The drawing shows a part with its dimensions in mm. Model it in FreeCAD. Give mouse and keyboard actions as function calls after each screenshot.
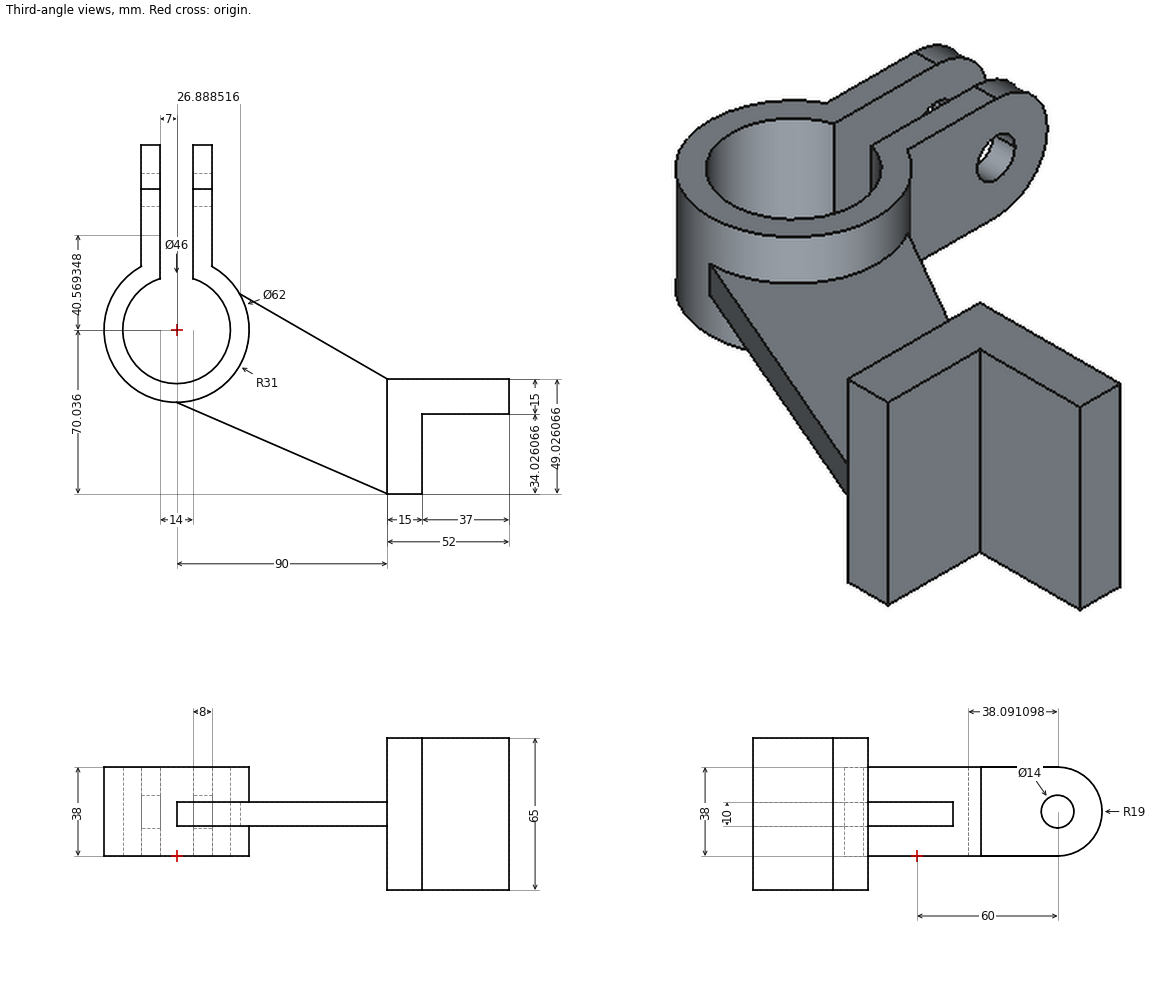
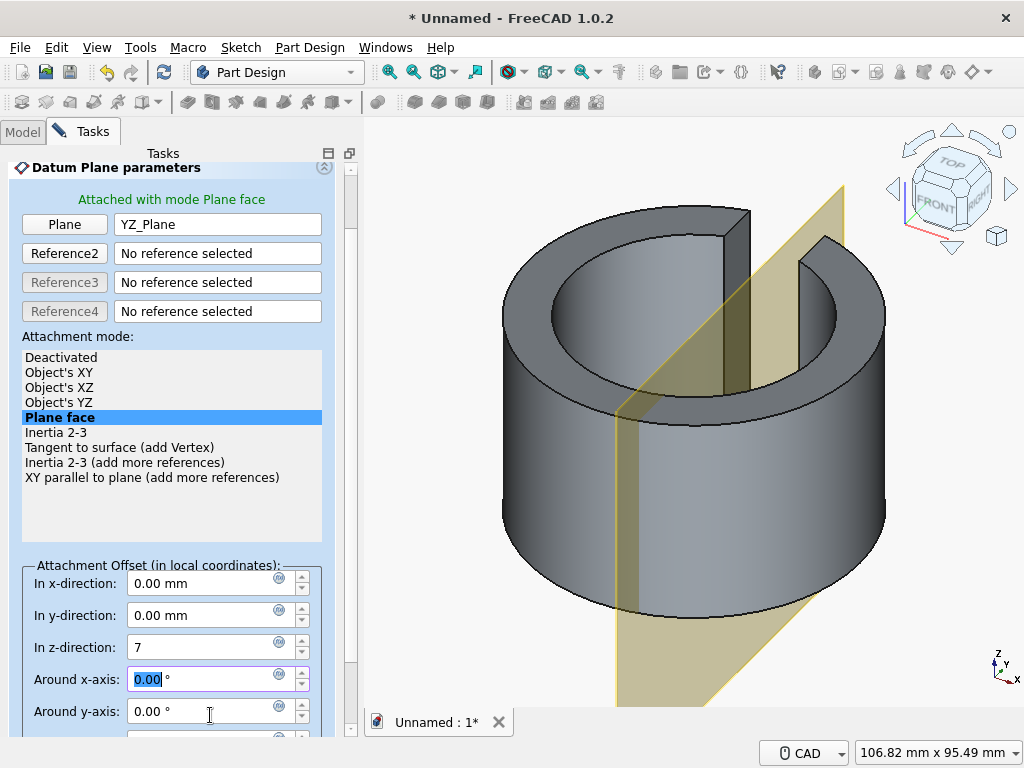
scroll(351, 450, up, 2)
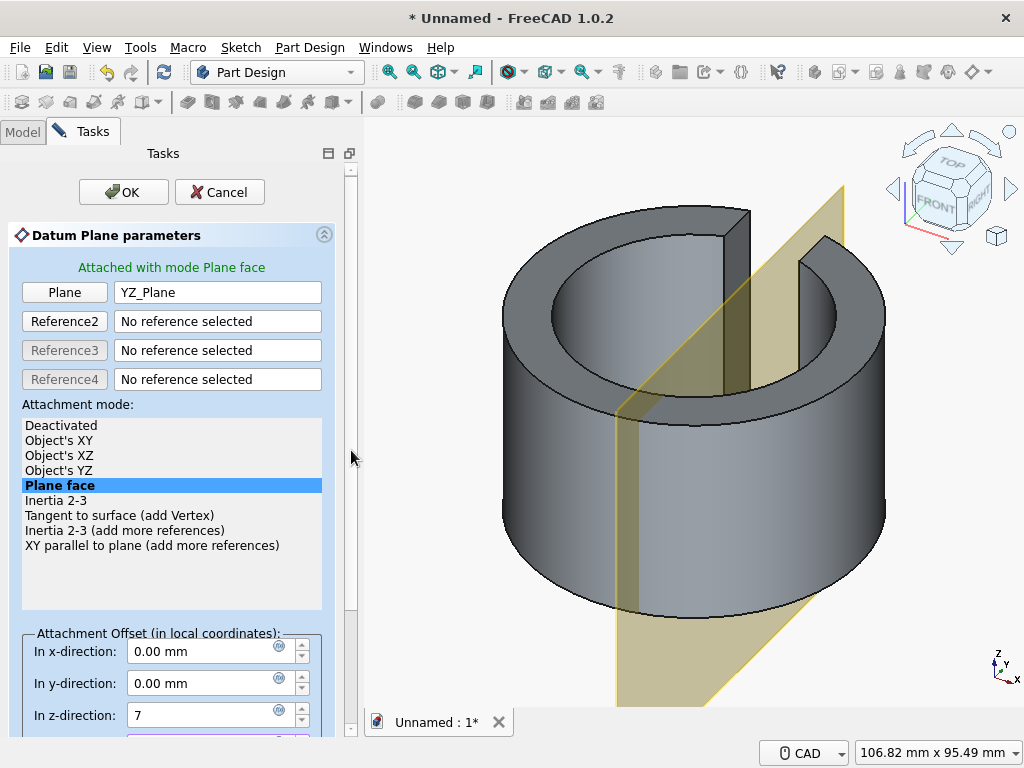
click(124, 192)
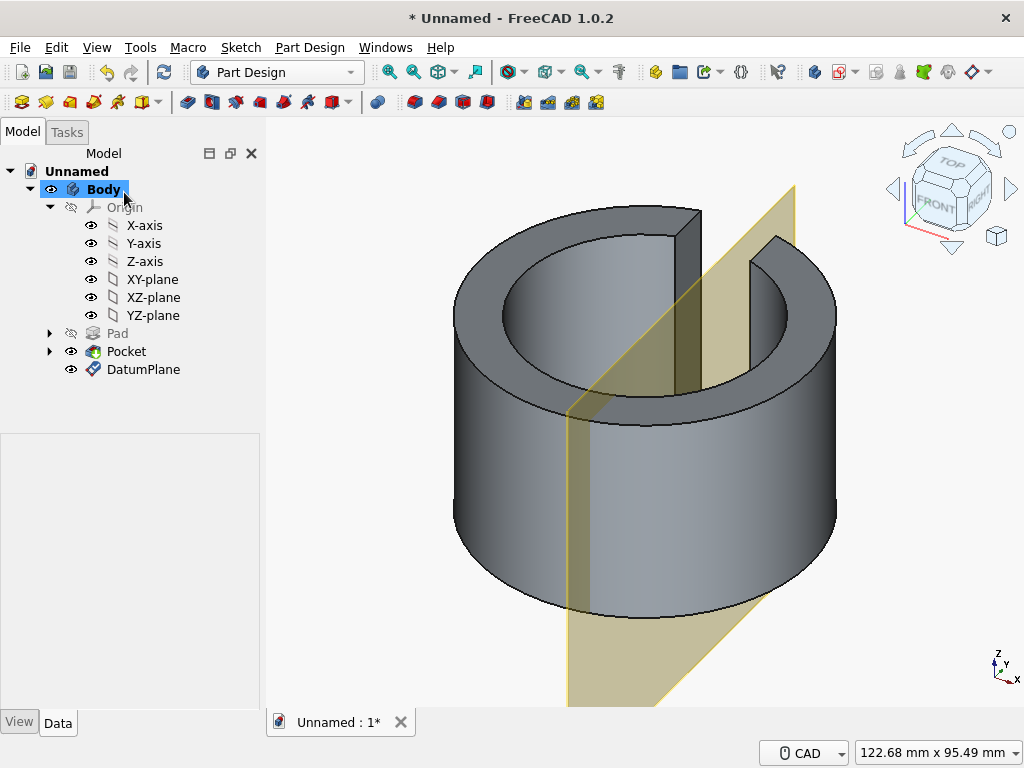
click(116, 369)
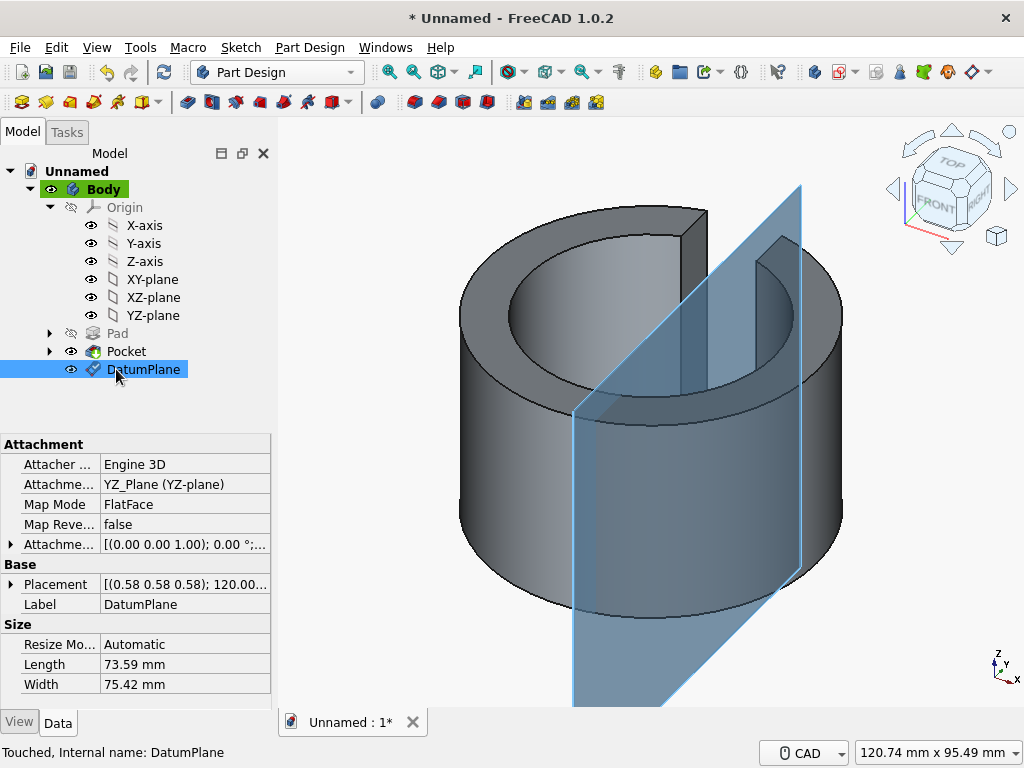
click(840, 72)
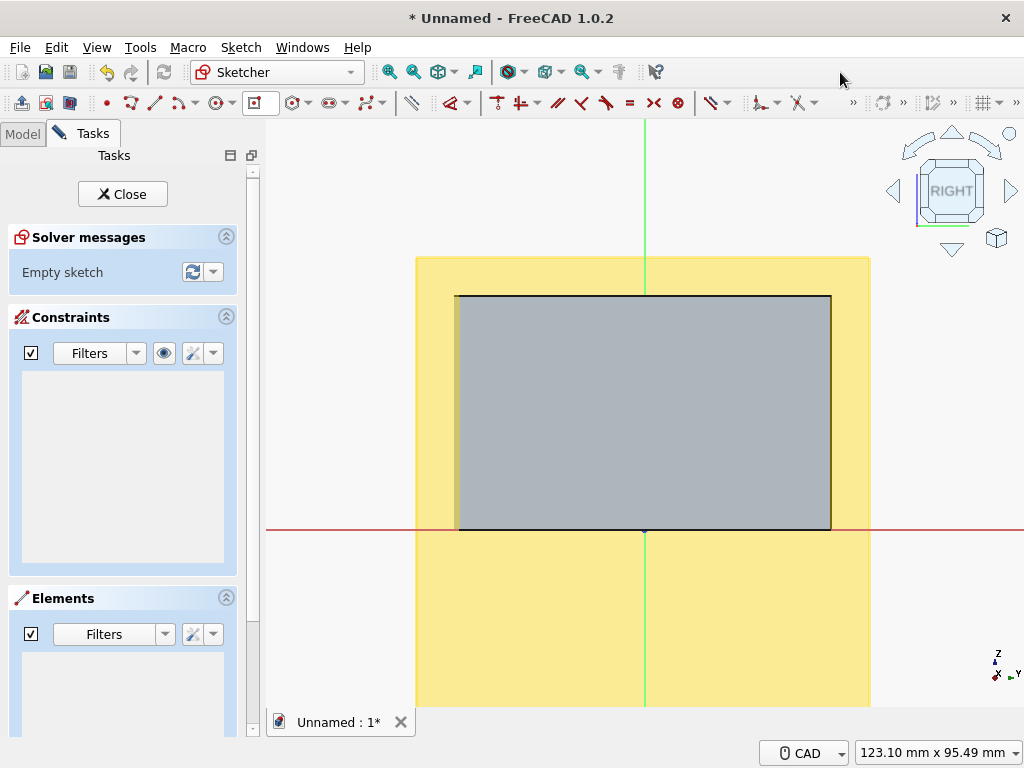
key(q)
key(s)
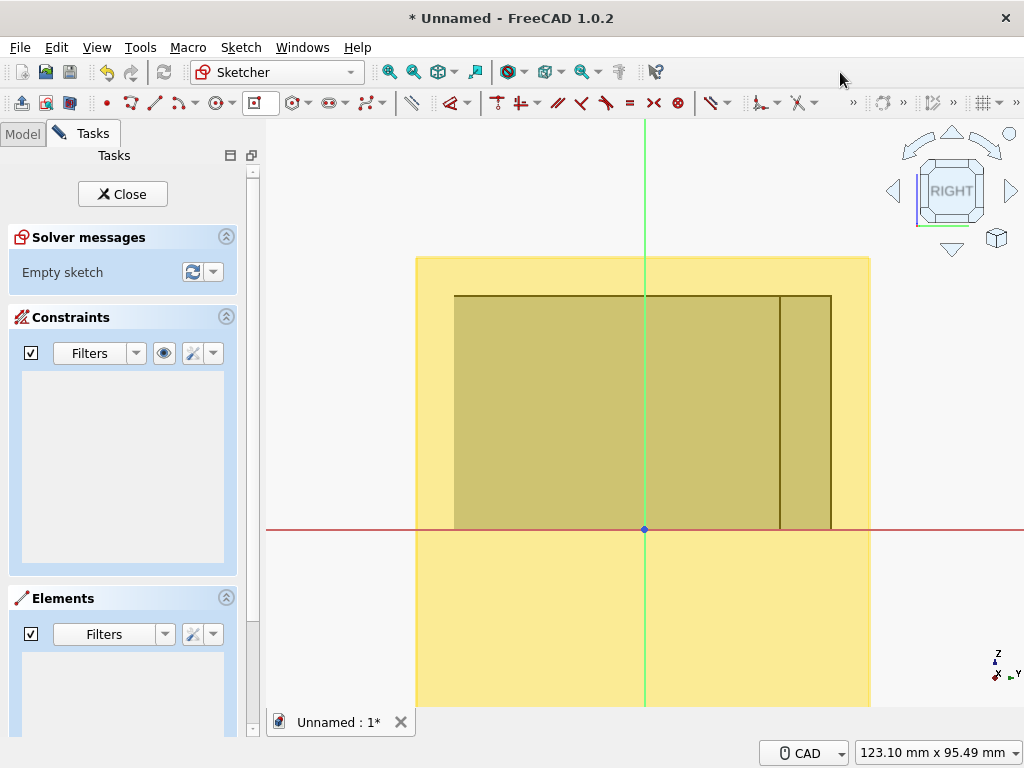
scroll(294, 413, down, 3)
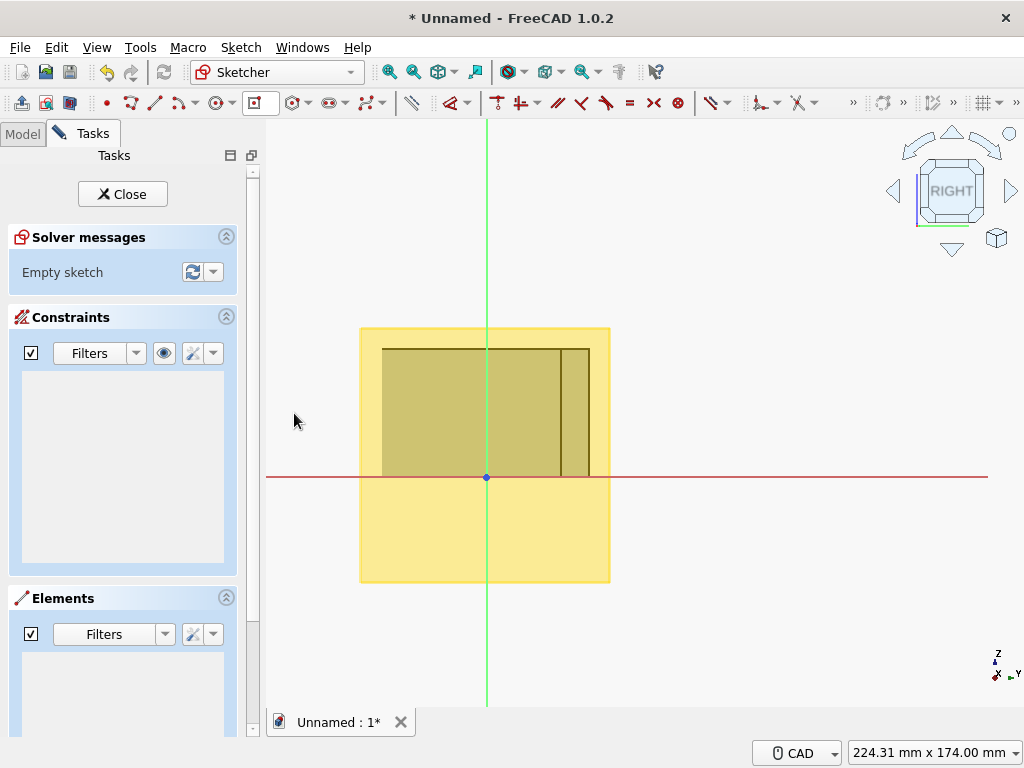
scroll(709, 414, up, 2)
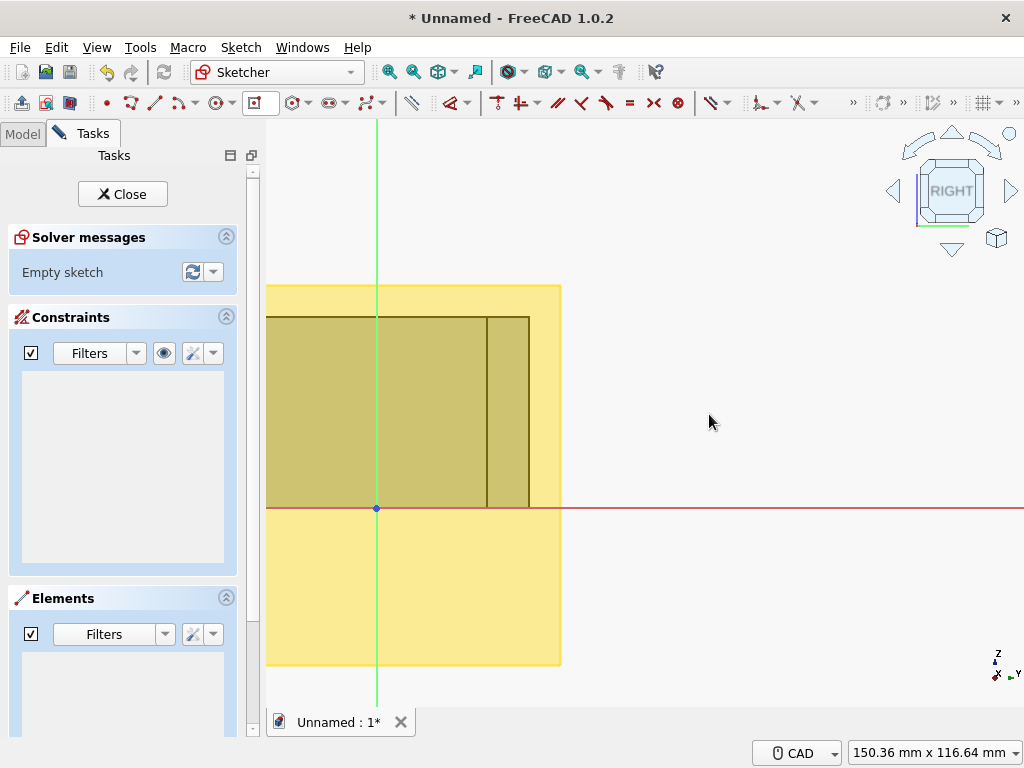
click(132, 104)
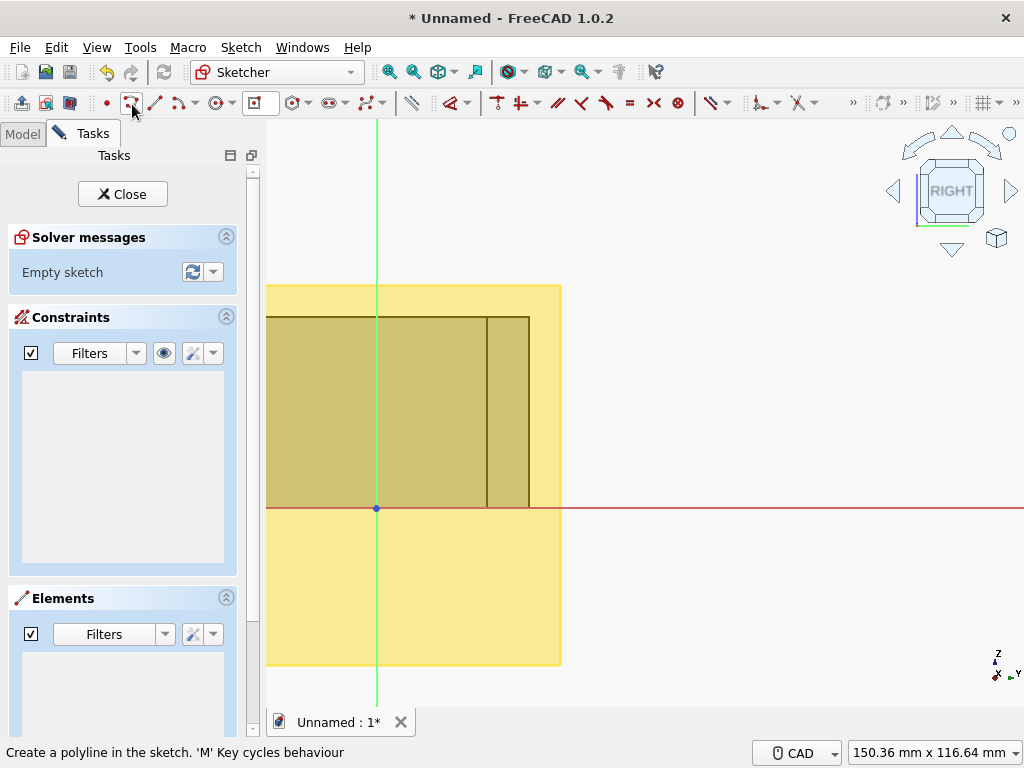
click(679, 317)
click(487, 317)
click(487, 508)
click(679, 499)
right_click(679, 499)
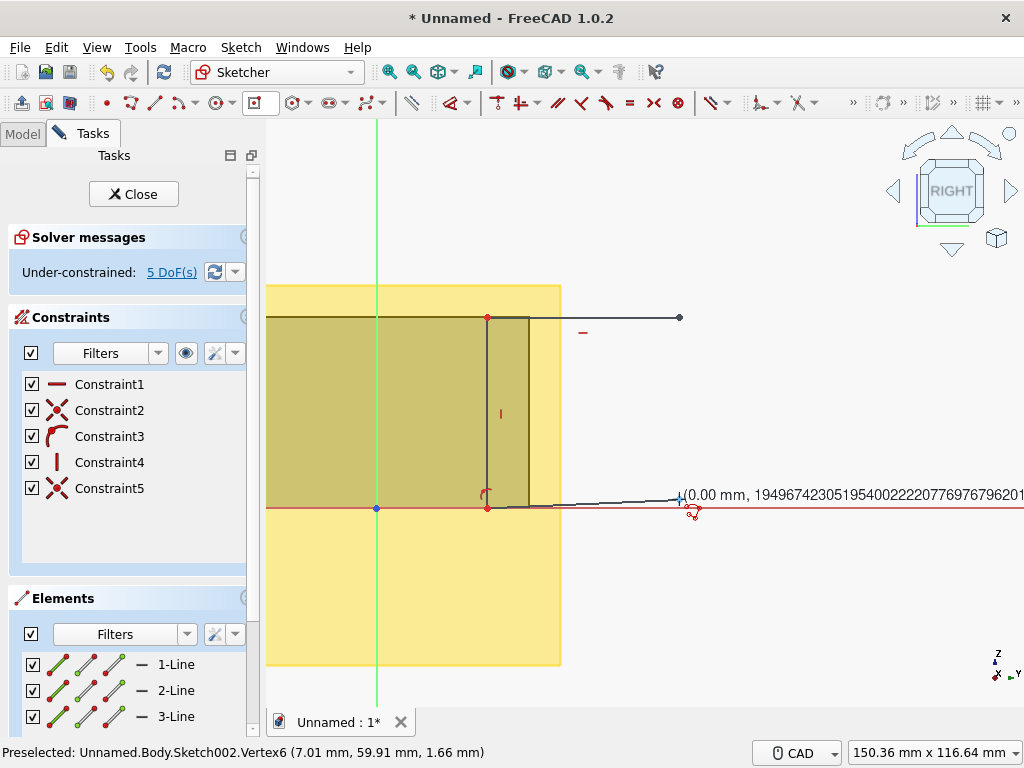
key(g)
key(3)
key(a)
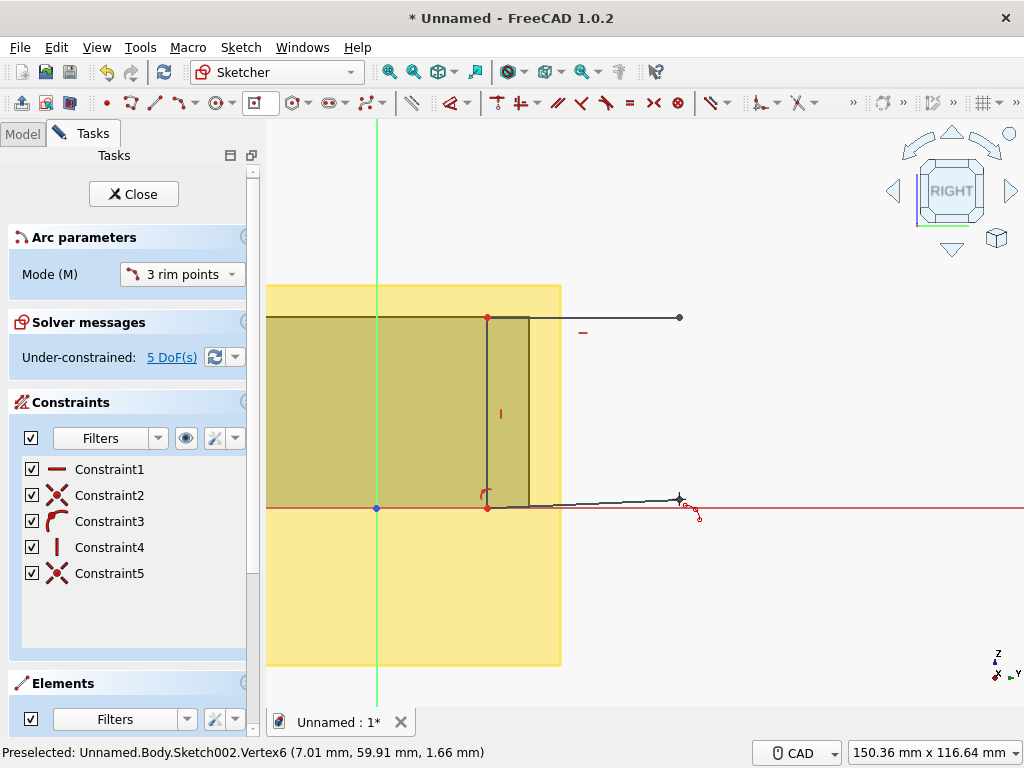
click(679, 500)
click(679, 318)
click(775, 413)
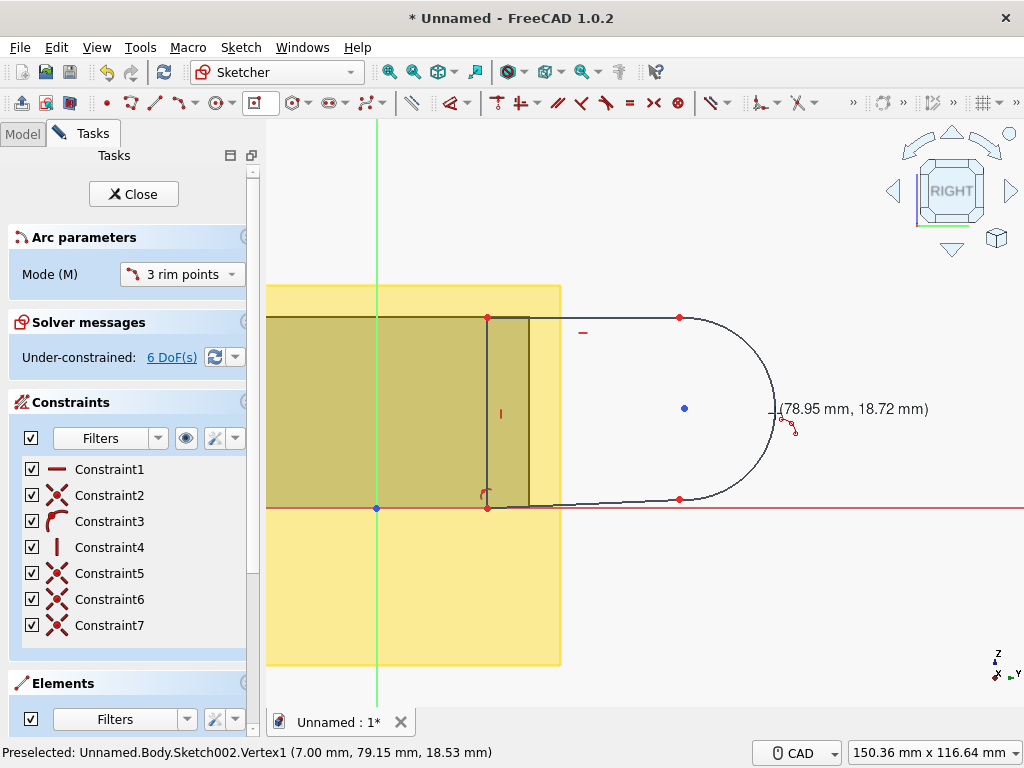
key(g)
key(c)